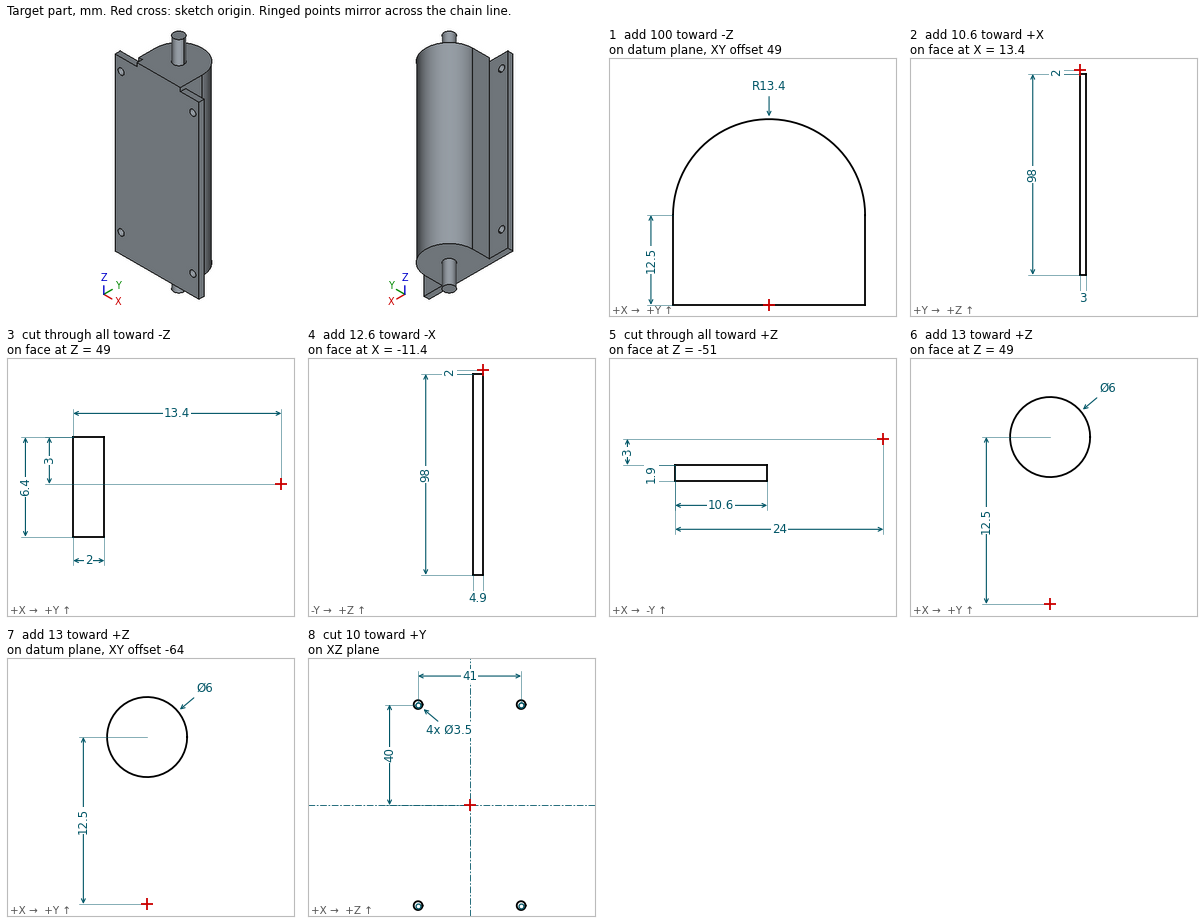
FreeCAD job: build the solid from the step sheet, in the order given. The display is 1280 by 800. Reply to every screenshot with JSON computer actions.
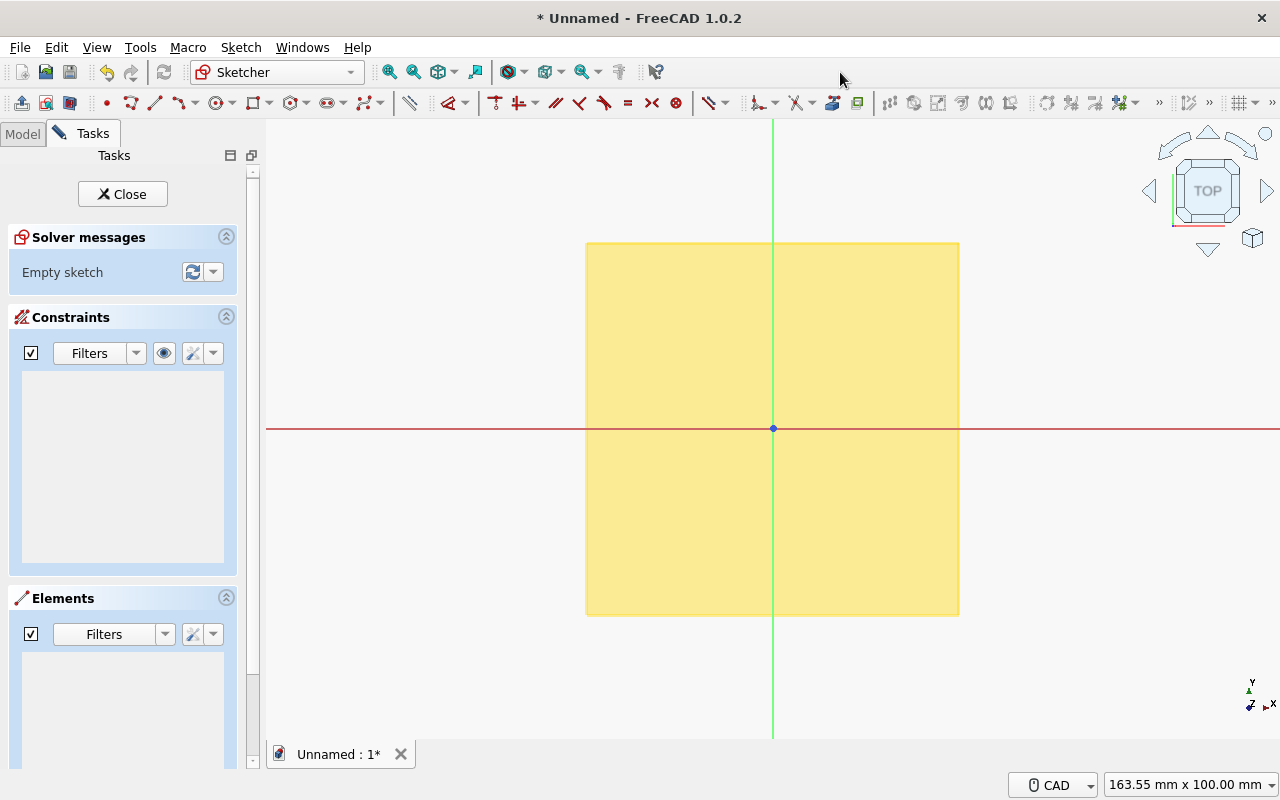
{"action": "scroll", "coordinate": [813, 302], "scroll_direction": "up", "scroll_amount": 5}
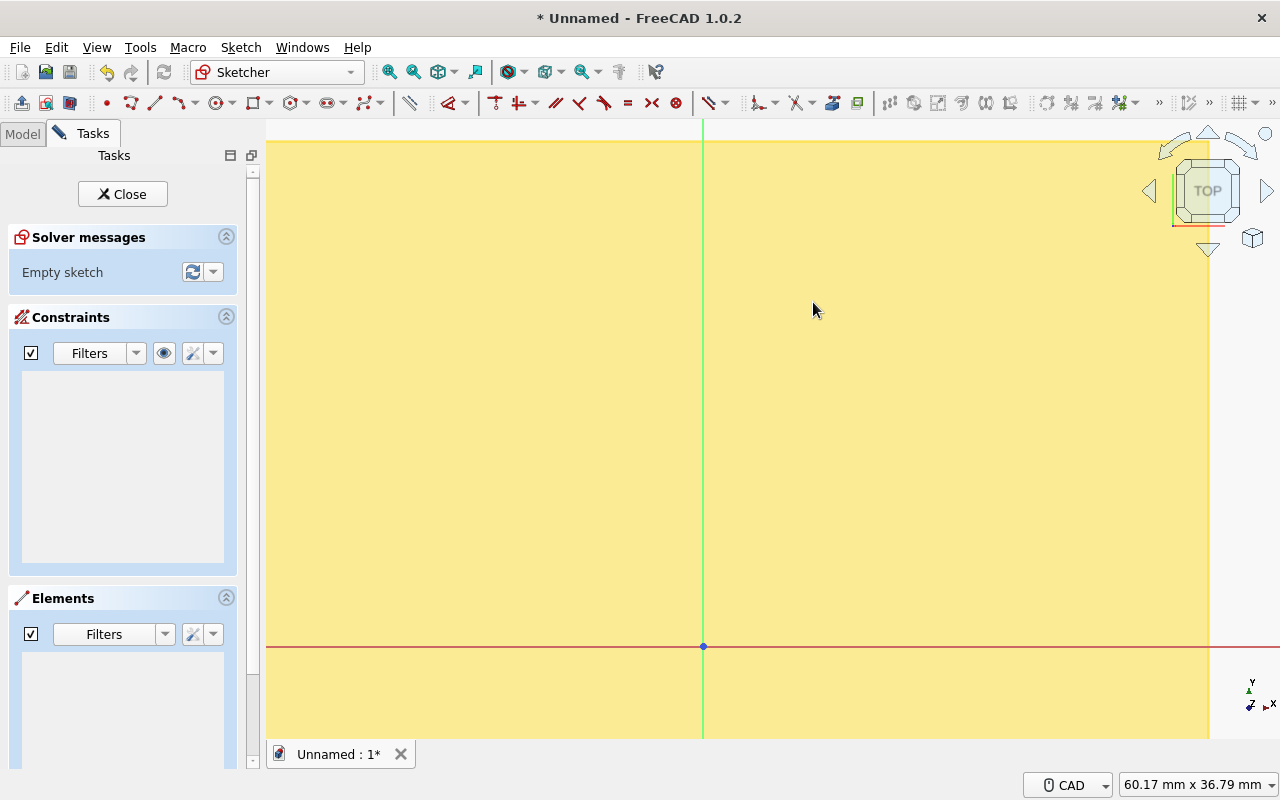
{"action": "left_click", "coordinate": [132, 104]}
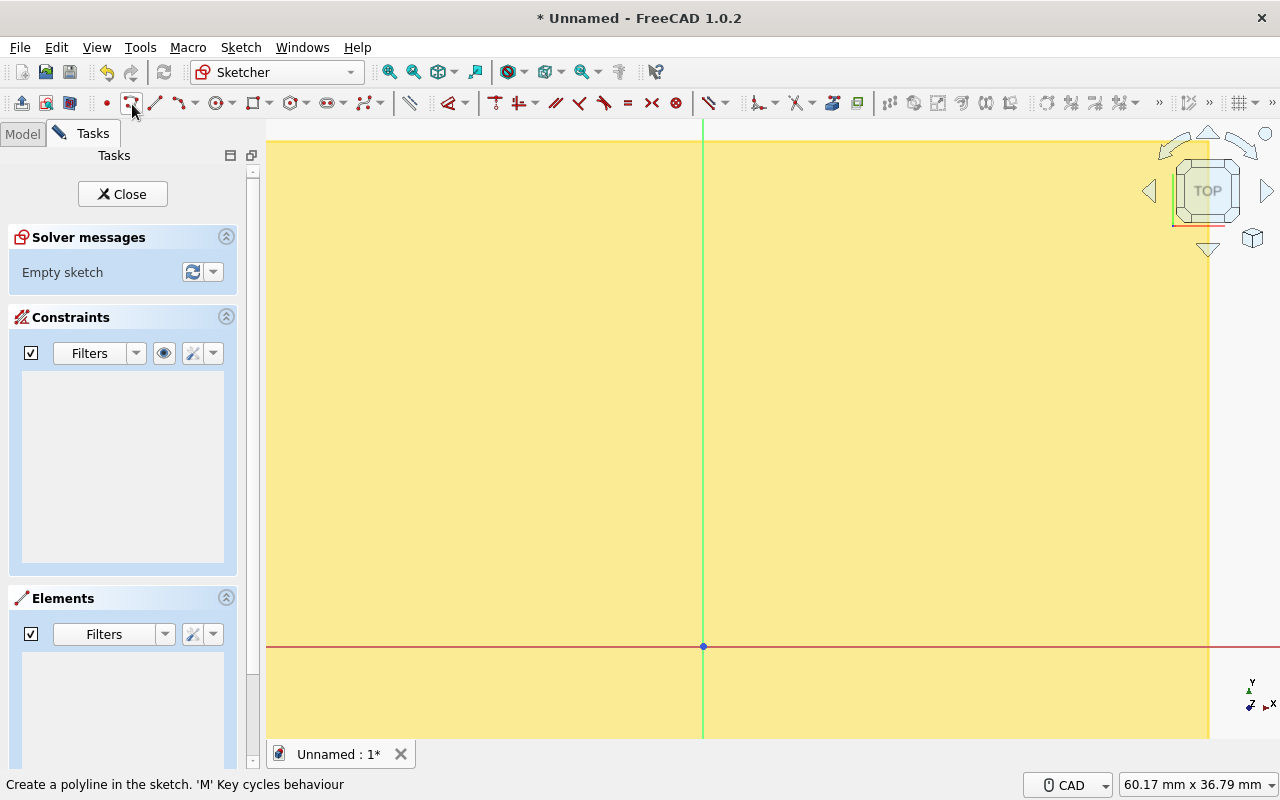
{"action": "left_click", "coordinate": [478, 436]}
{"action": "left_click", "coordinate": [478, 647]}
{"action": "left_click", "coordinate": [929, 638]}
{"action": "left_click", "coordinate": [929, 436]}
{"action": "right_click", "coordinate": [929, 436]}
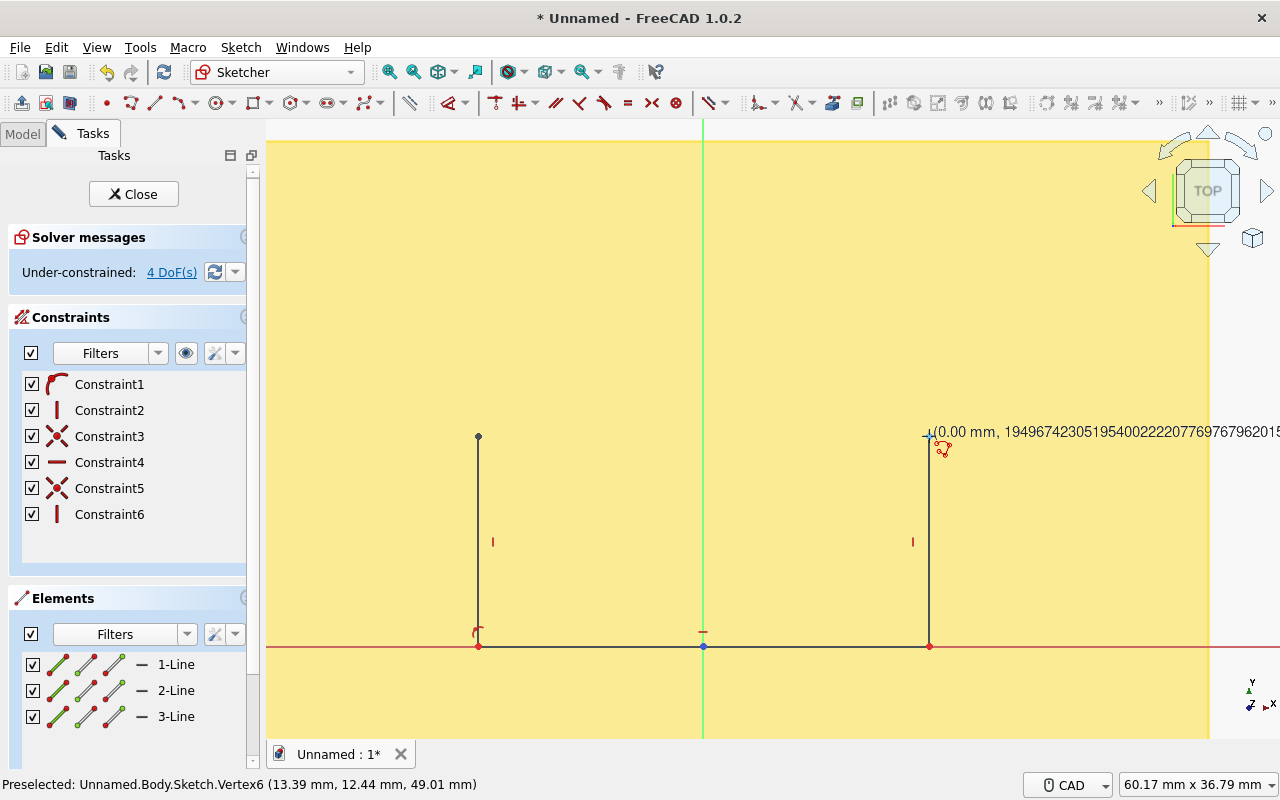
{"action": "left_click", "coordinate": [180, 104]}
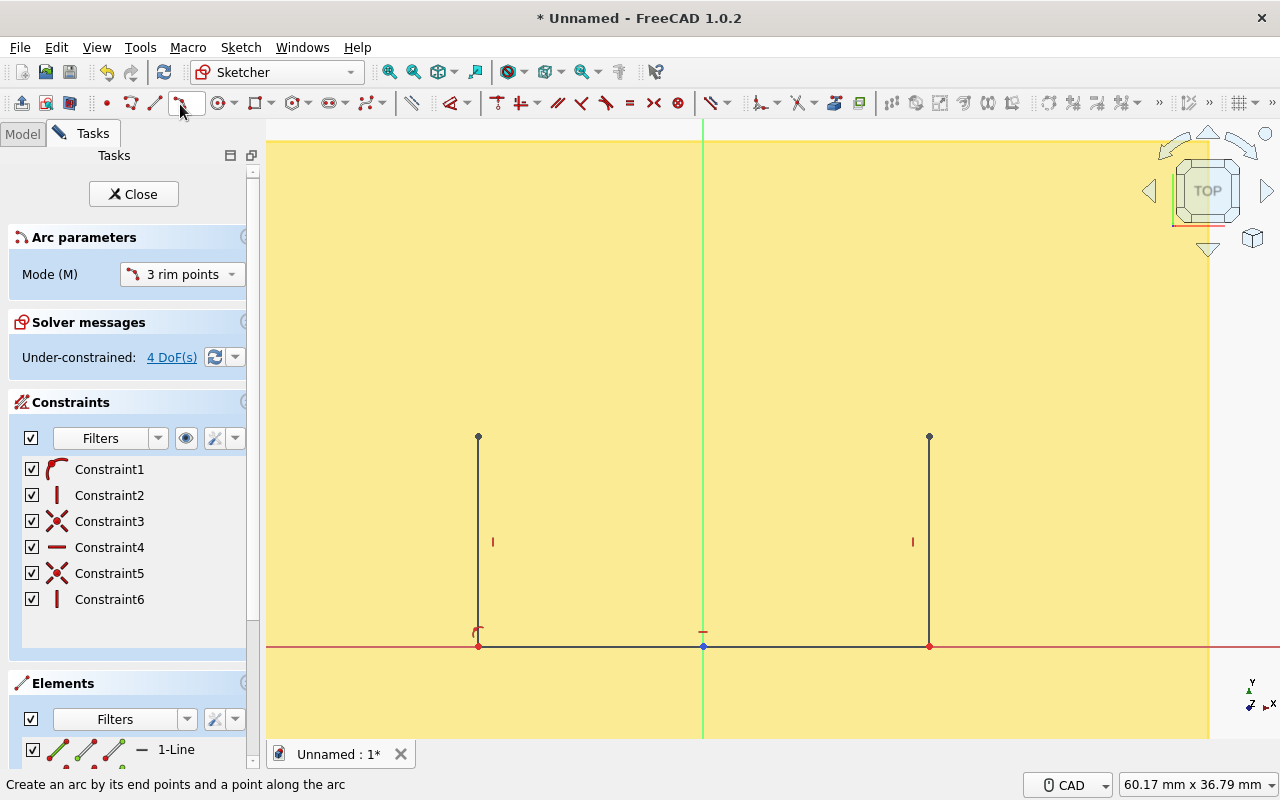
{"action": "left_click", "coordinate": [929, 437]}
{"action": "left_click", "coordinate": [478, 437]}
{"action": "left_click", "coordinate": [773, 221]}
{"action": "key", "text": "Escape"}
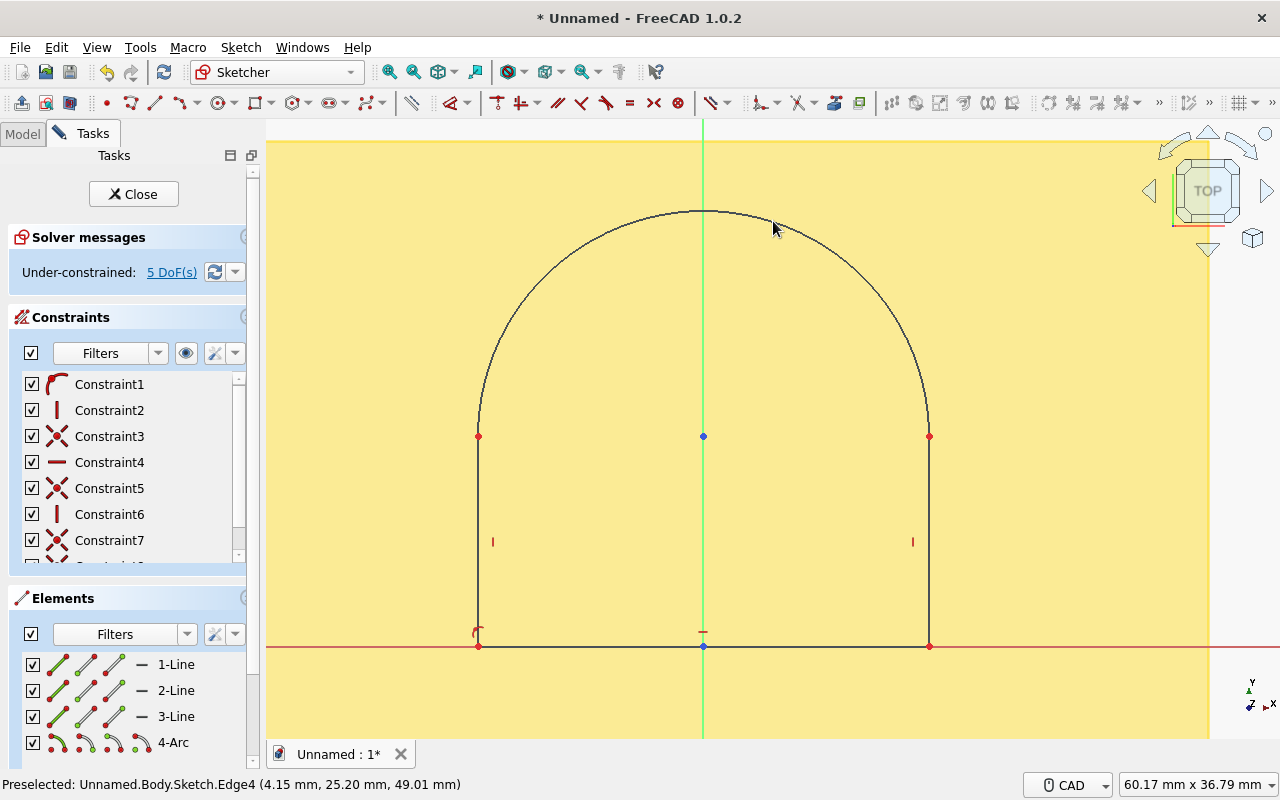
{"action": "left_click", "coordinate": [478, 500]}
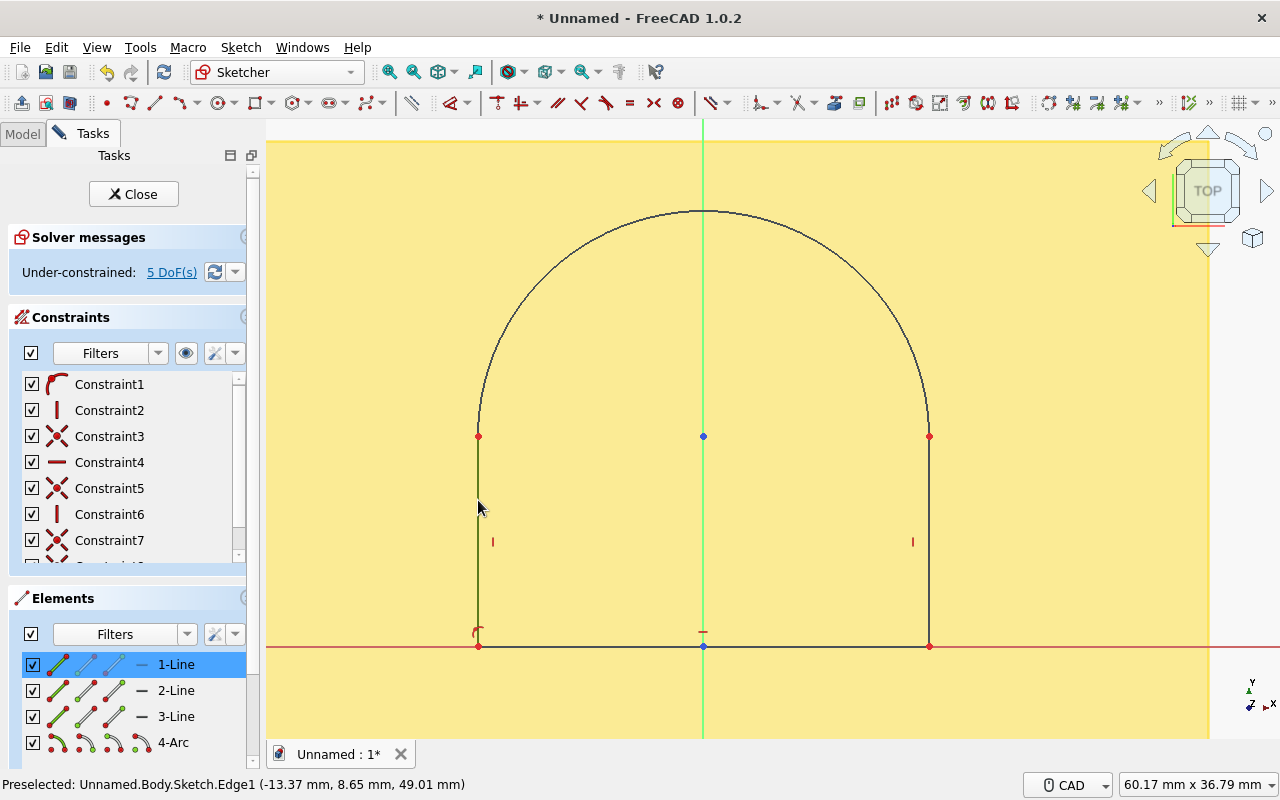
{"action": "left_click", "coordinate": [836, 254]}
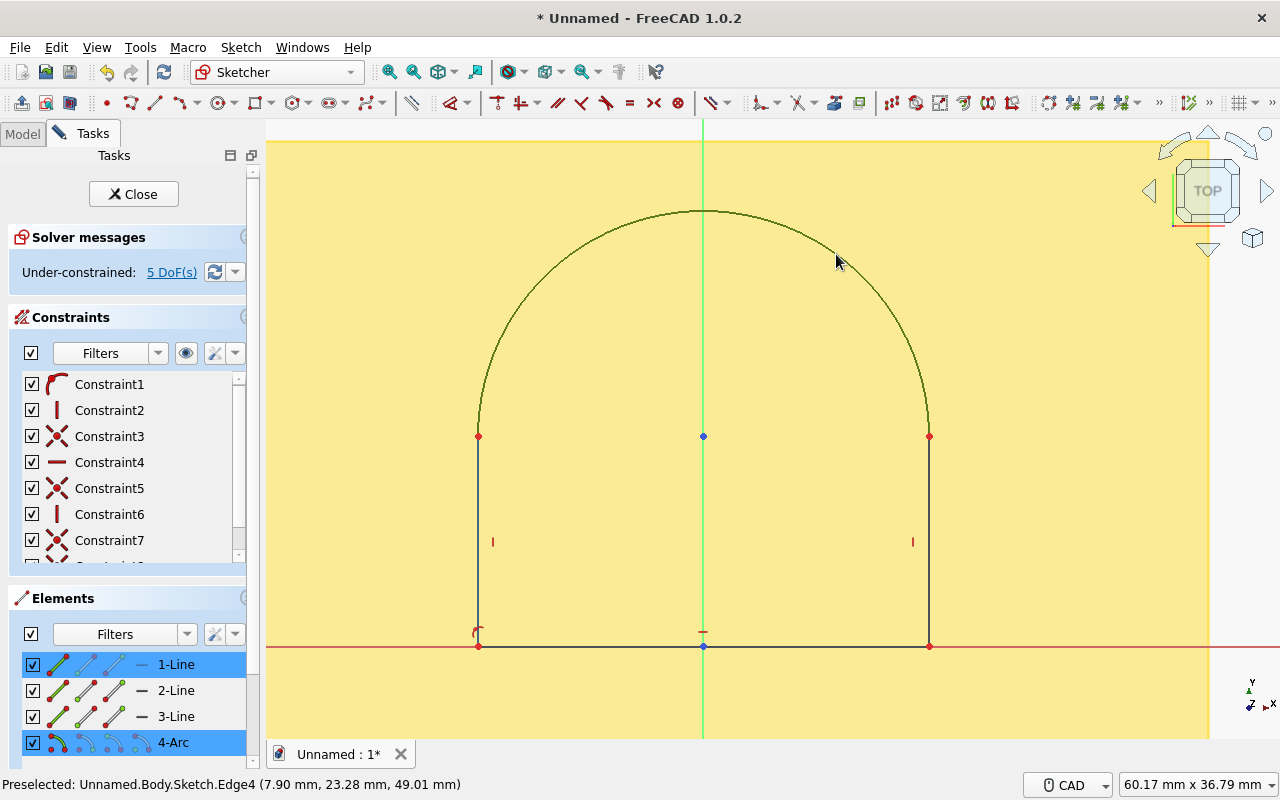
{"action": "left_click", "coordinate": [606, 104]}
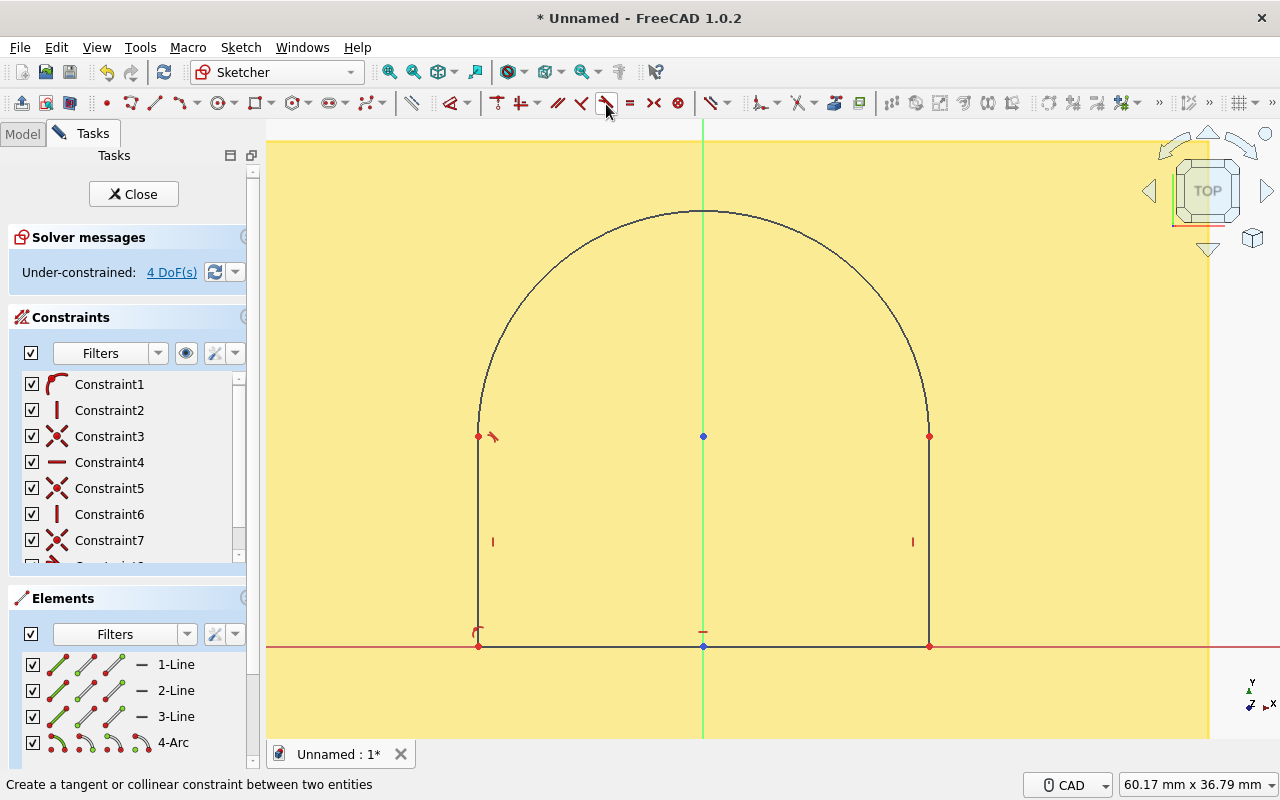
{"action": "left_click", "coordinate": [929, 584]}